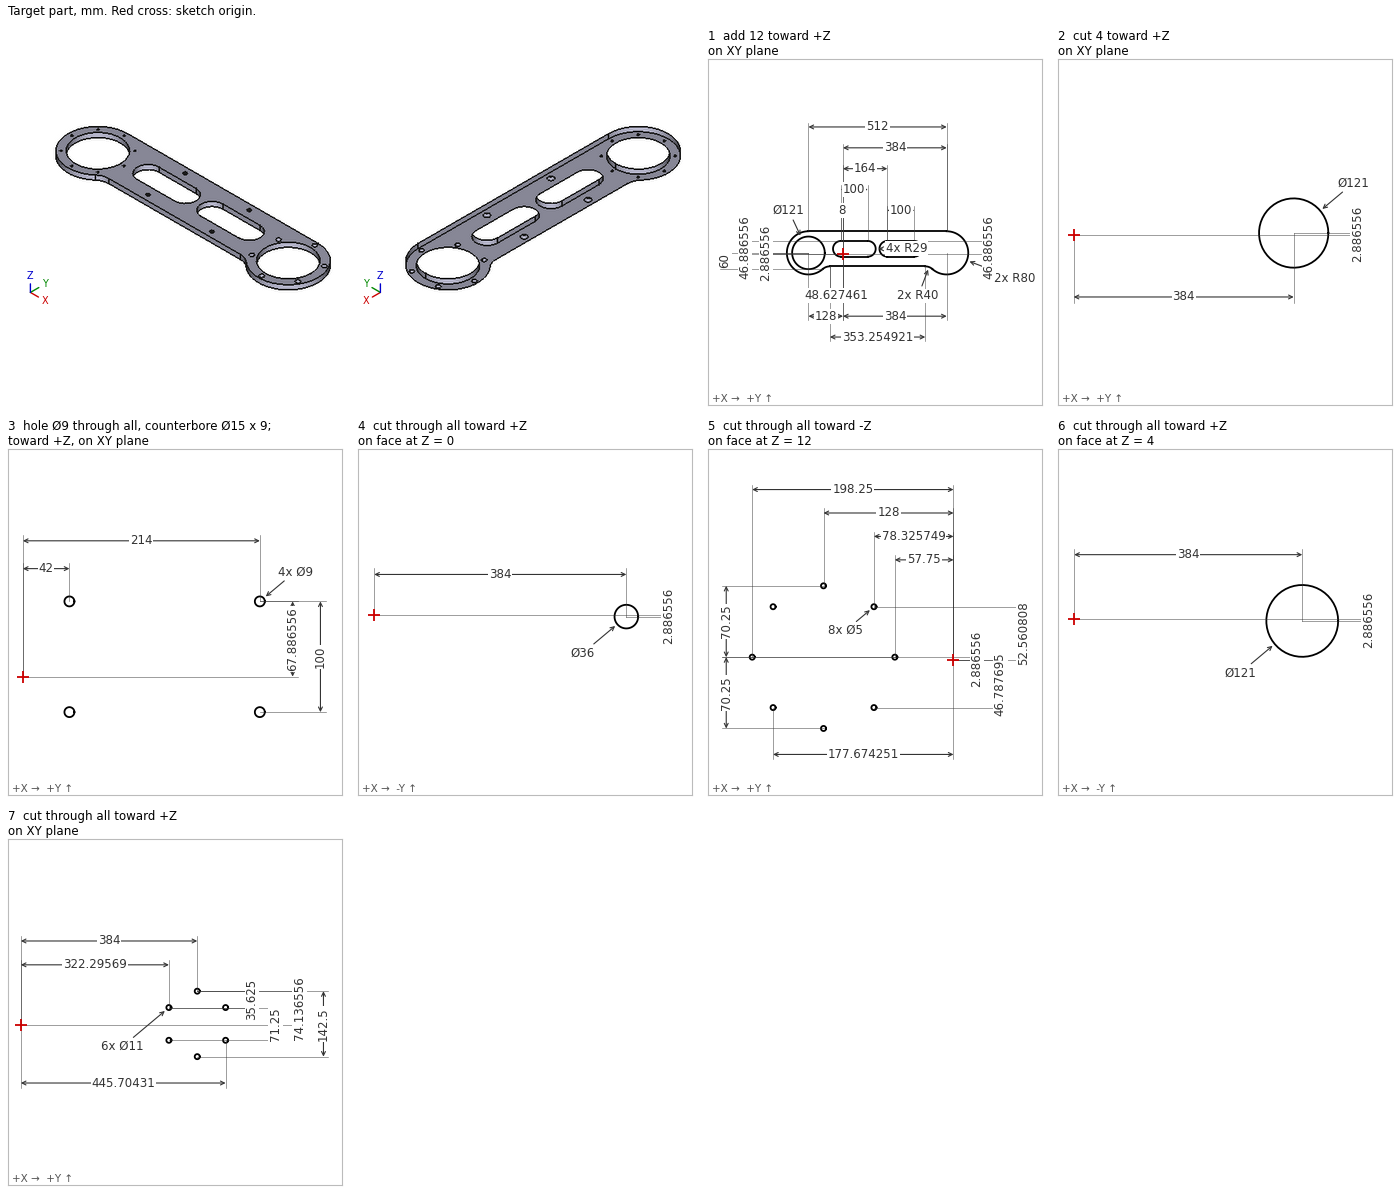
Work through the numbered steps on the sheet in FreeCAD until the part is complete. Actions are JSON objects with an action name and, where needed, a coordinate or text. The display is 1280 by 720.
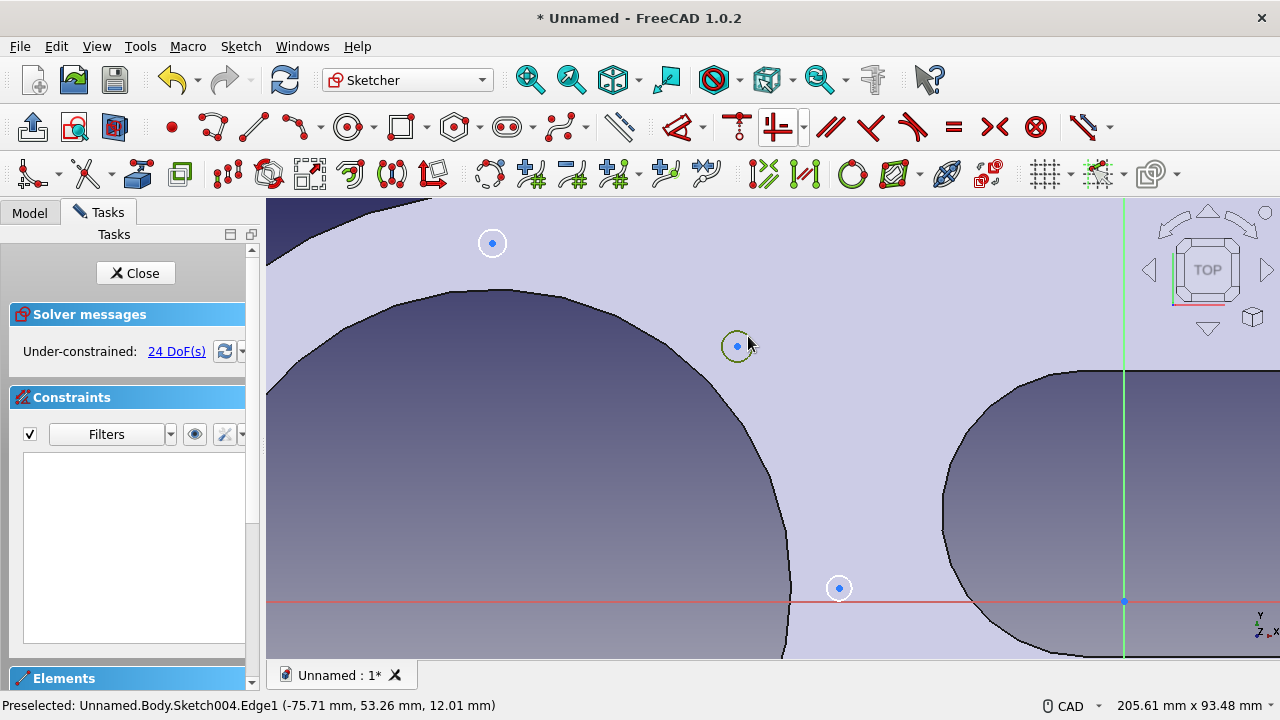
{"action": "left_click", "coordinate": [502, 234]}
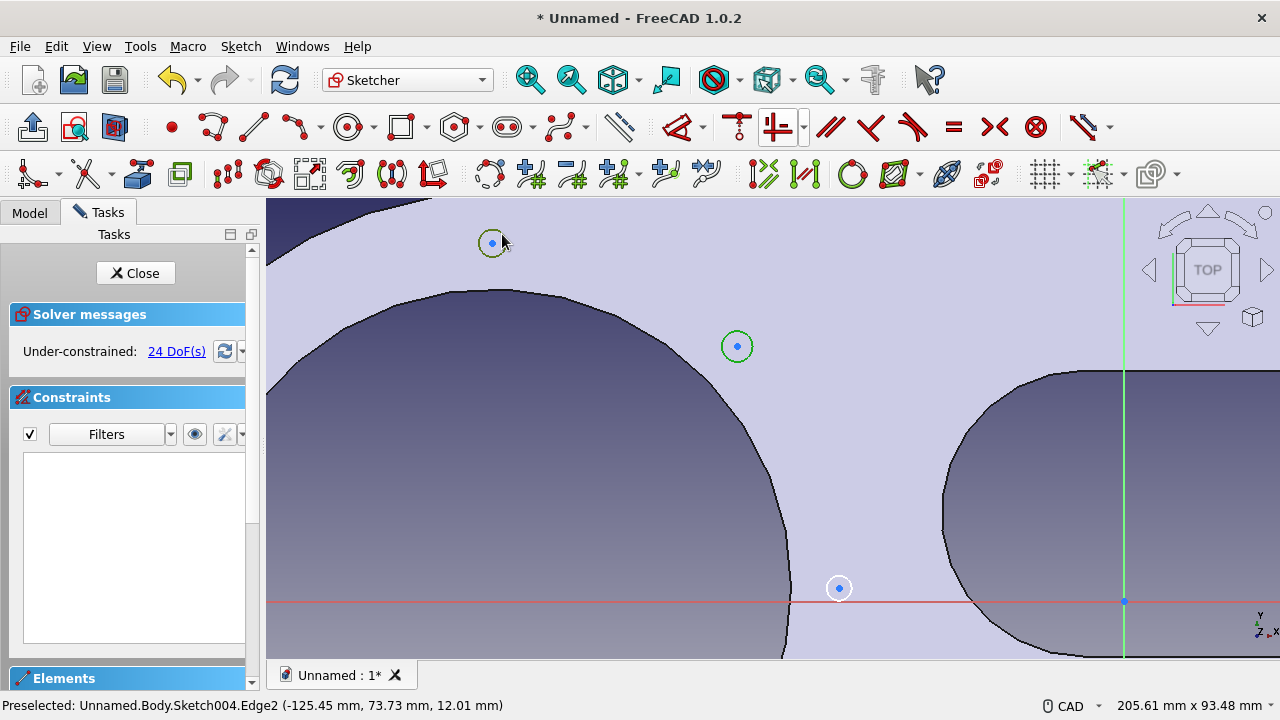
{"action": "left_click", "coordinate": [848, 580]}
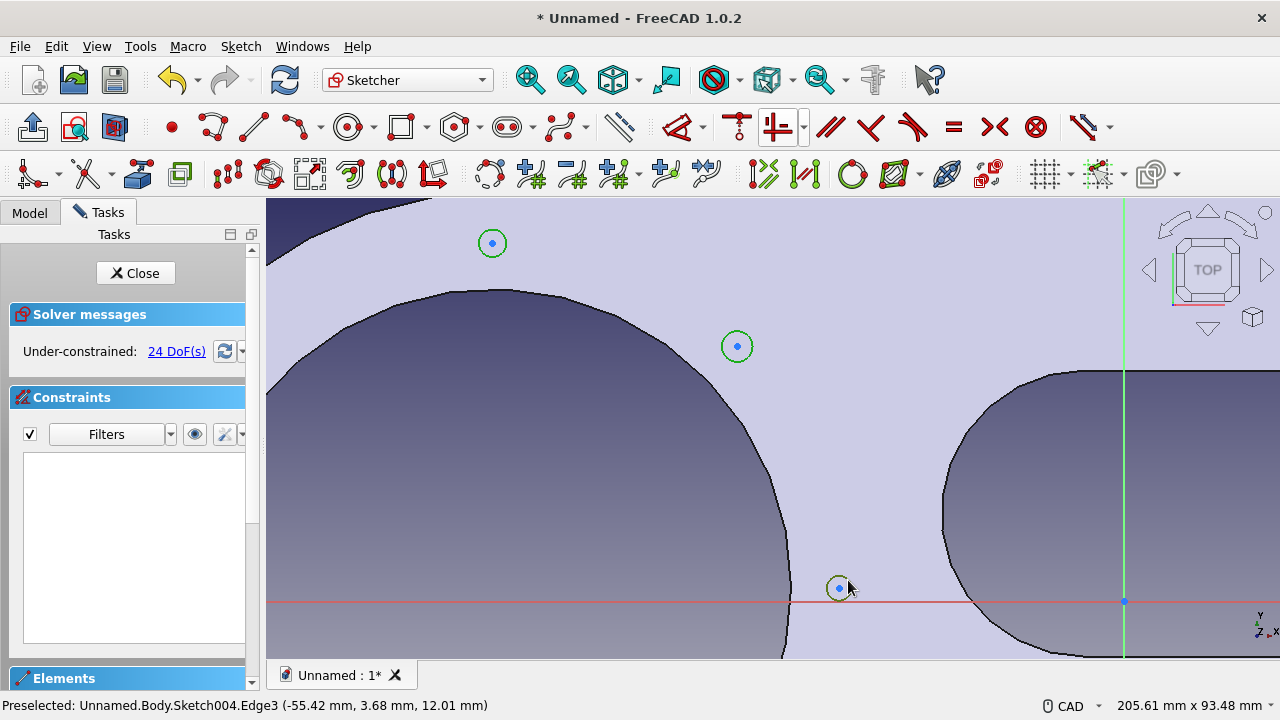
{"action": "scroll", "coordinate": [748, 336], "scroll_direction": "down", "scroll_amount": 5}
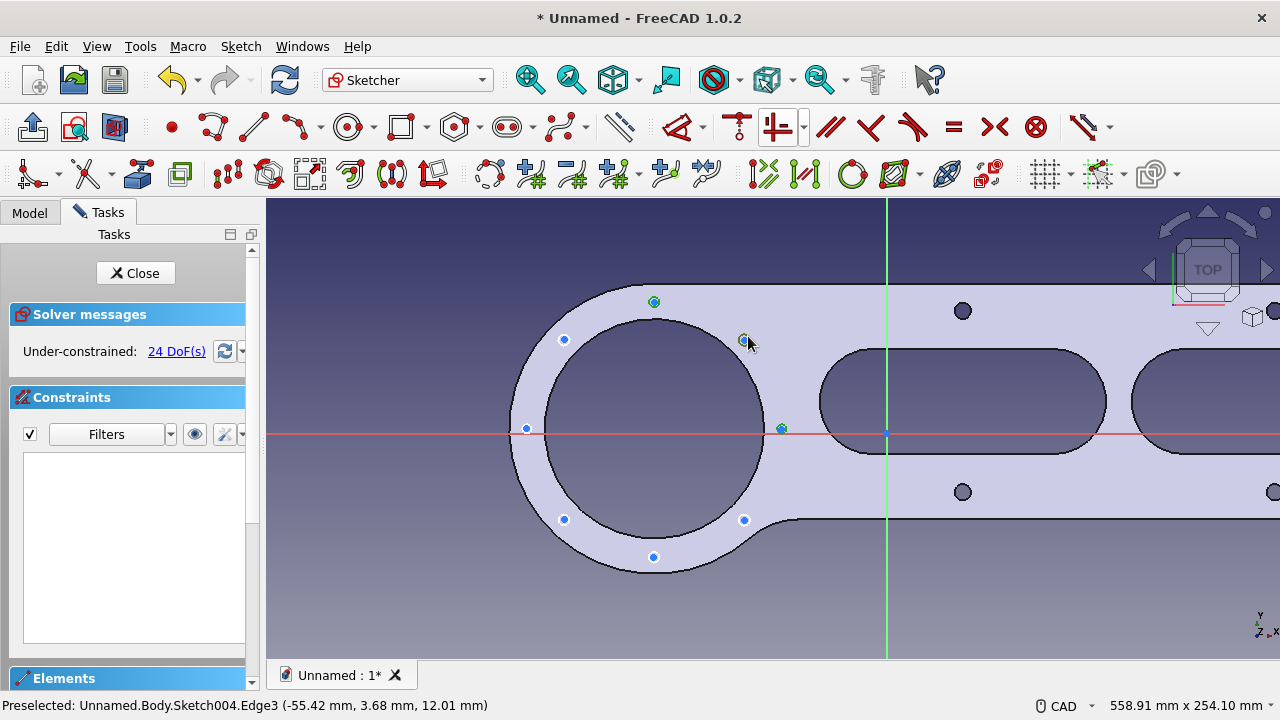
{"action": "scroll", "coordinate": [748, 516], "scroll_direction": "up", "scroll_amount": 5}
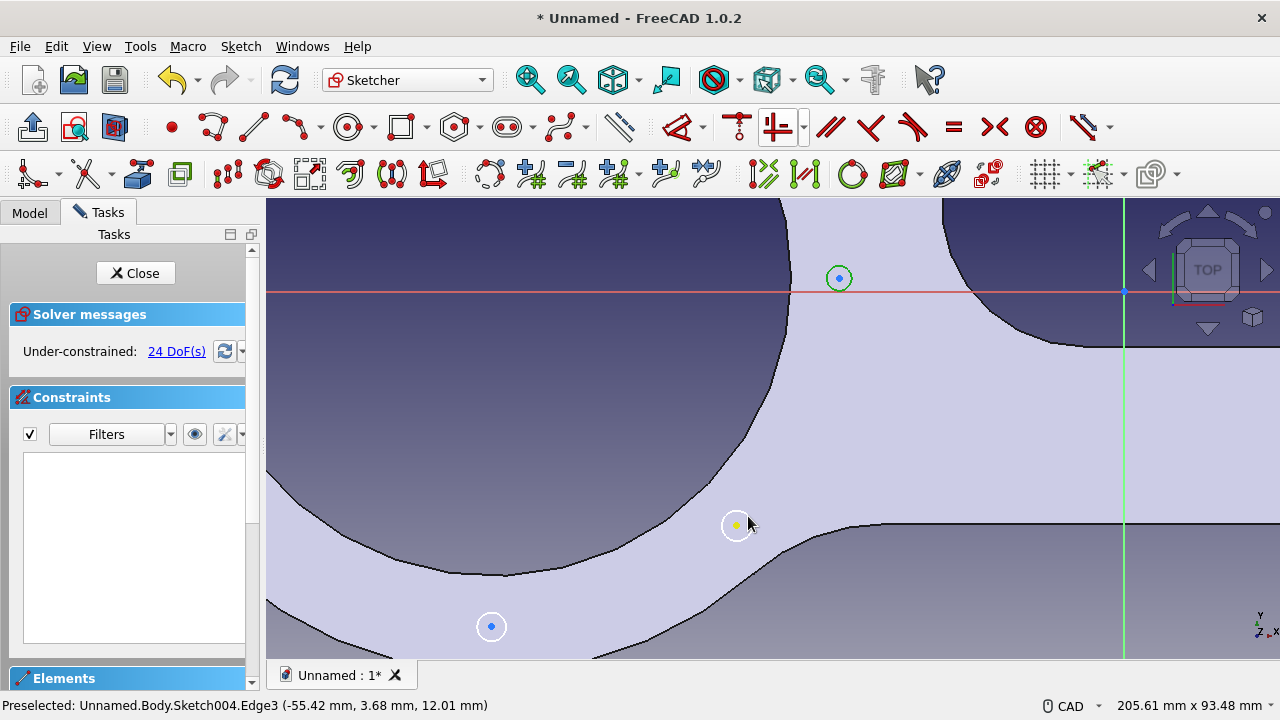
{"action": "left_click", "coordinate": [748, 515]}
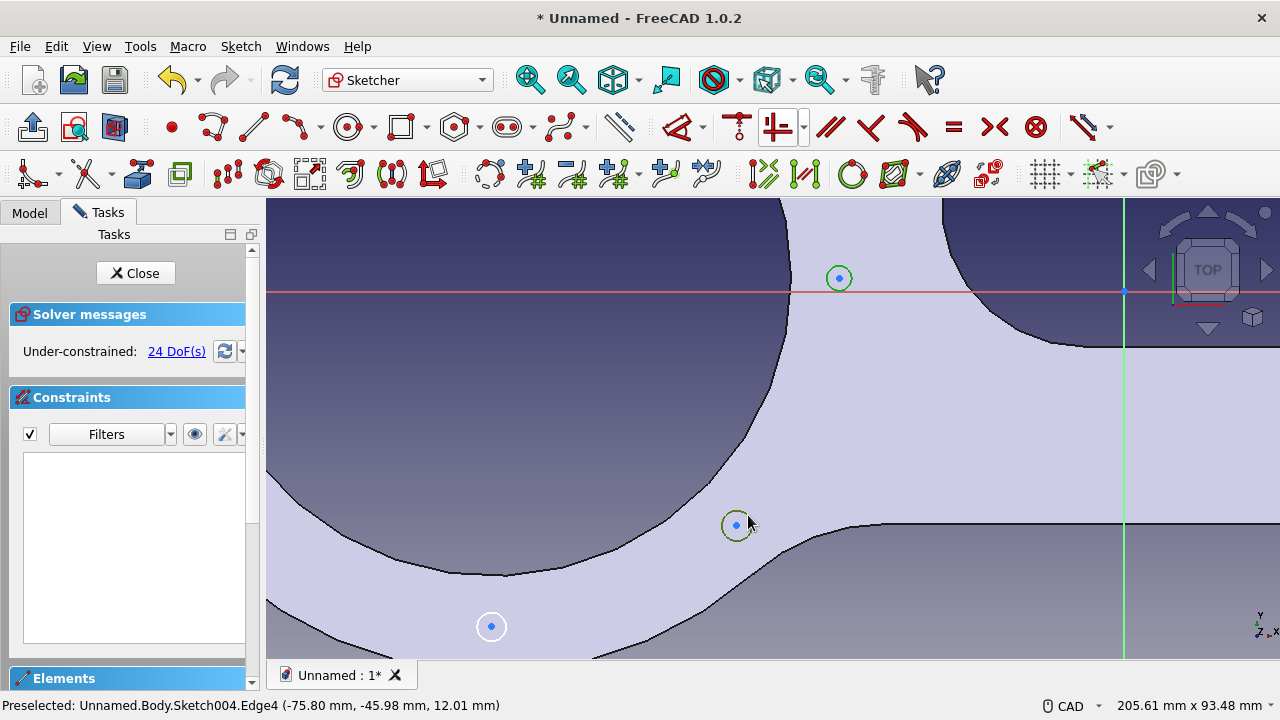
{"action": "left_click", "coordinate": [502, 617]}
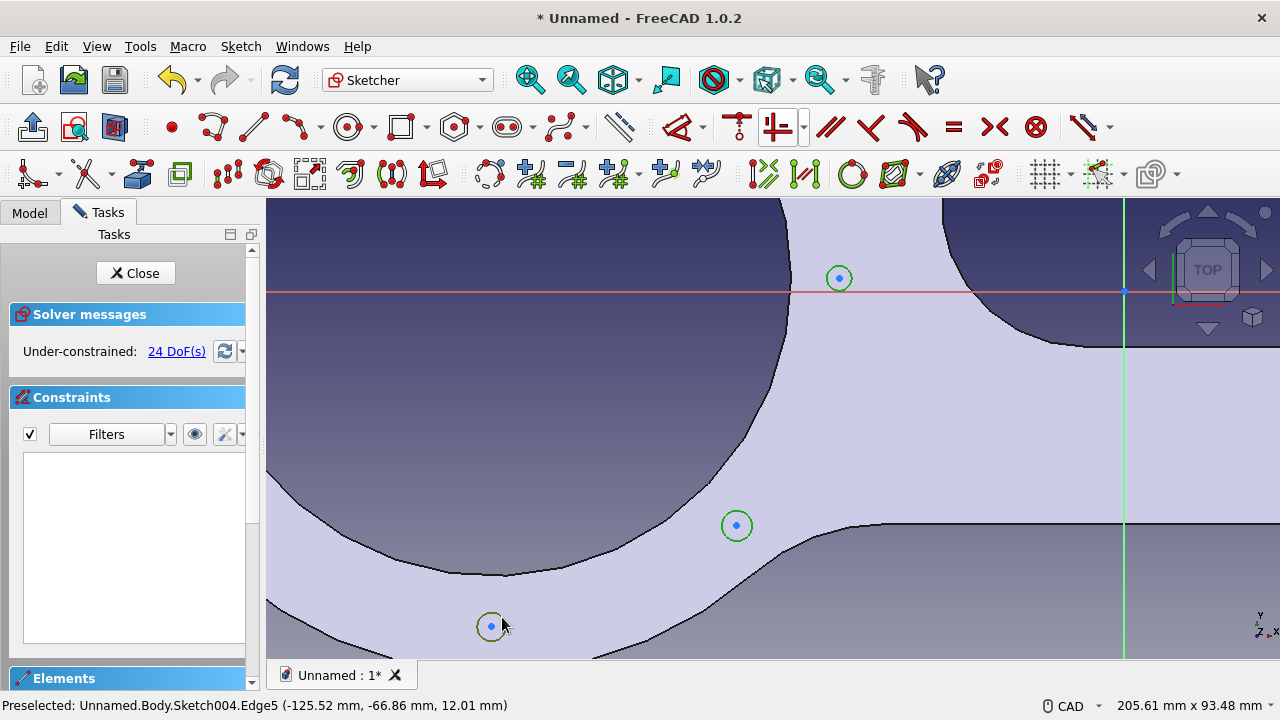
{"action": "scroll", "coordinate": [748, 516], "scroll_direction": "down", "scroll_amount": 5}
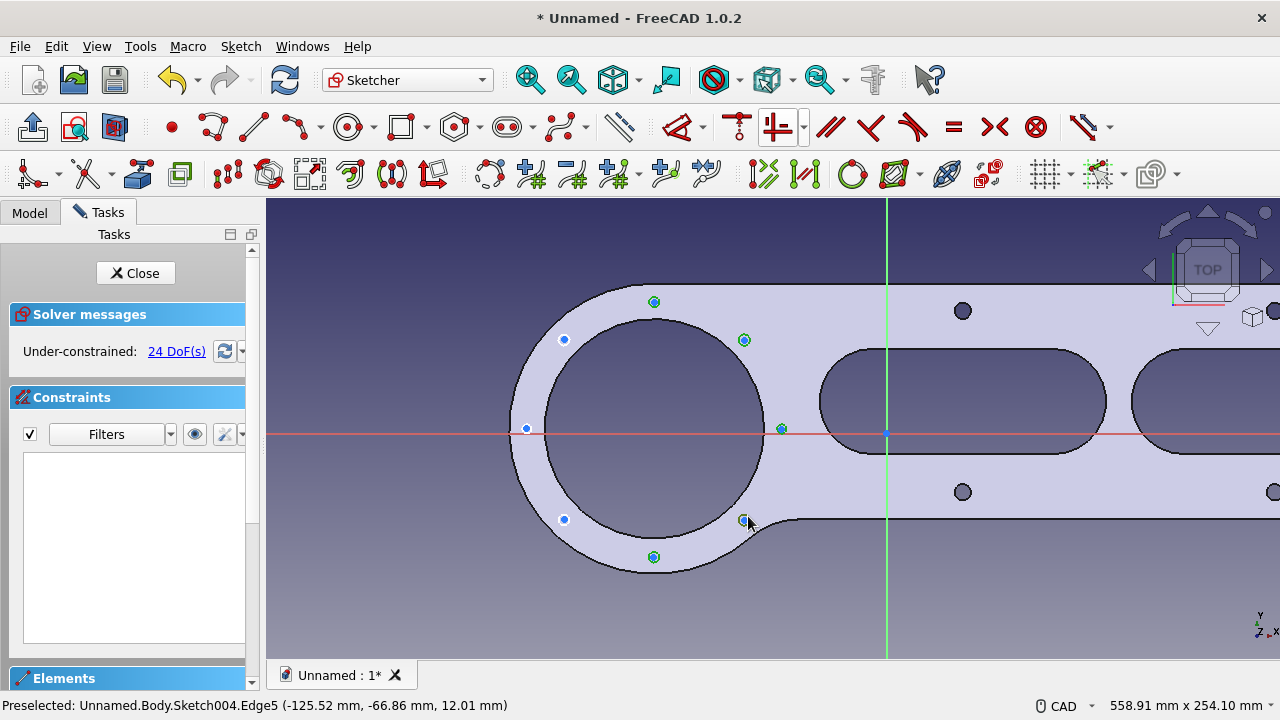
{"action": "scroll", "coordinate": [568, 516], "scroll_direction": "up", "scroll_amount": 5}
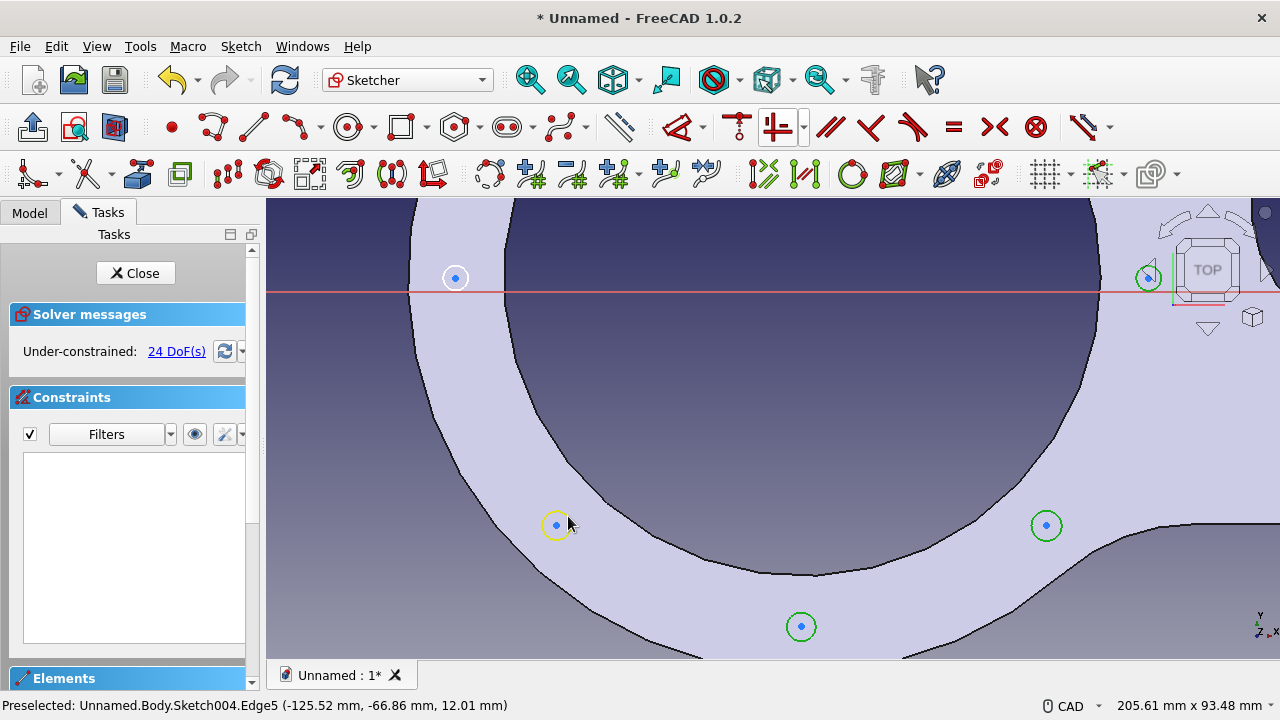
{"action": "left_click", "coordinate": [567, 516]}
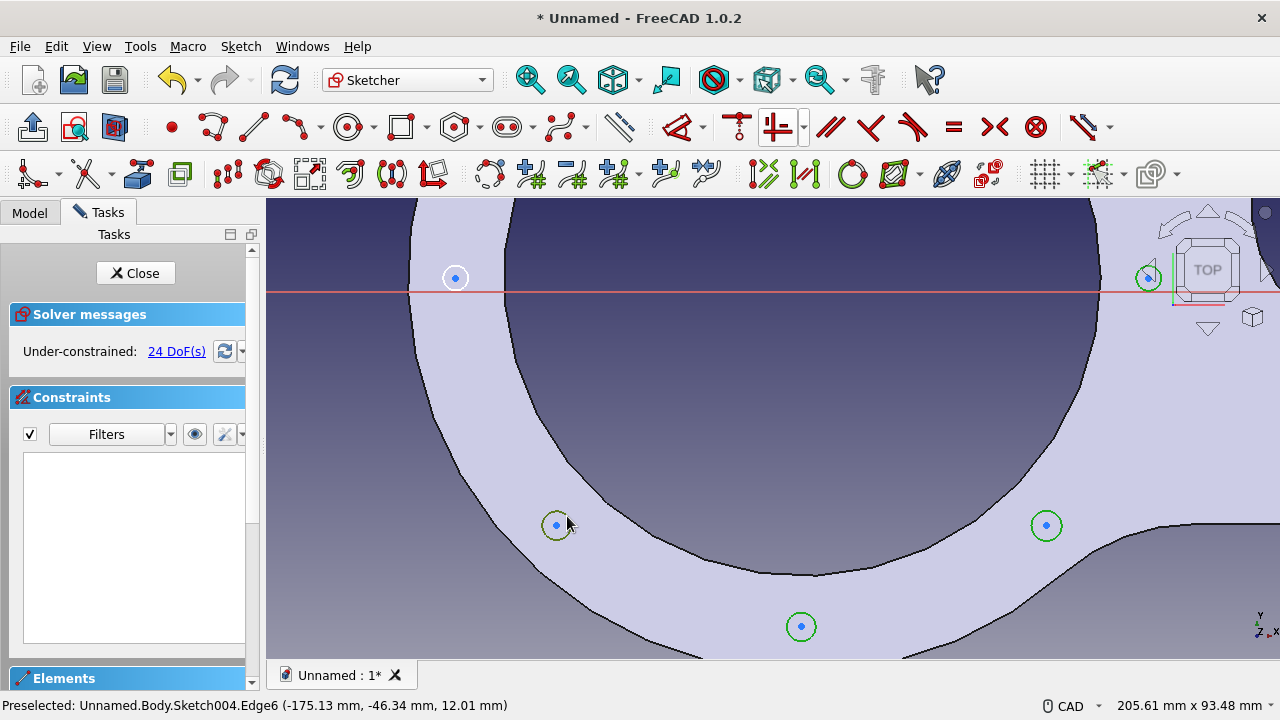
{"action": "left_click", "coordinate": [464, 269]}